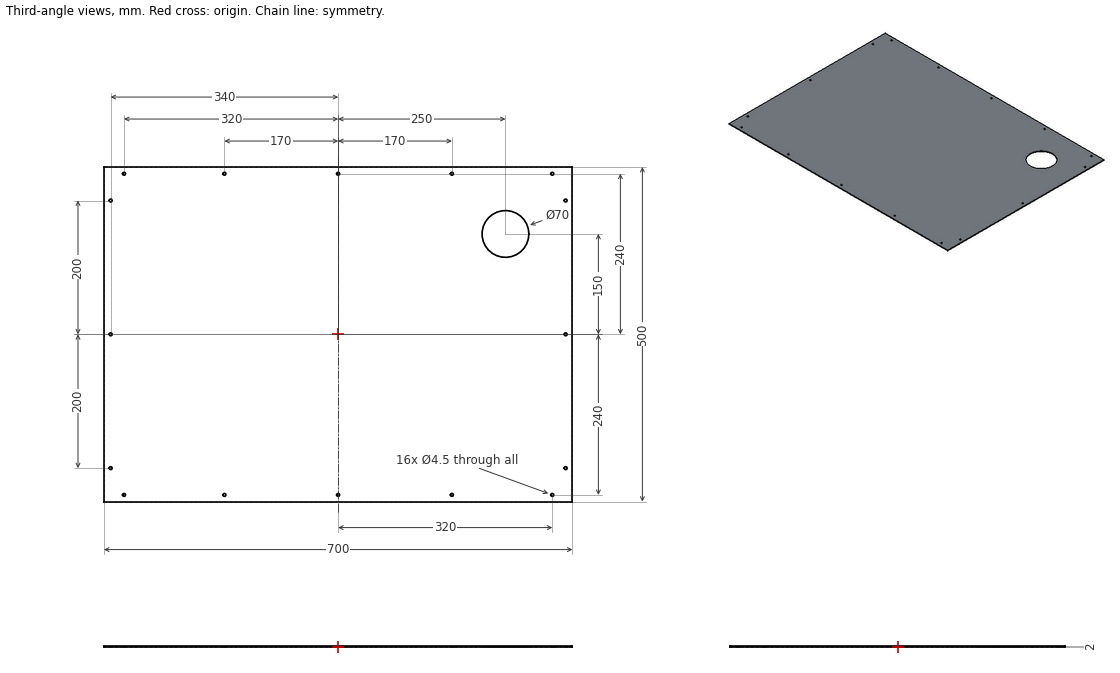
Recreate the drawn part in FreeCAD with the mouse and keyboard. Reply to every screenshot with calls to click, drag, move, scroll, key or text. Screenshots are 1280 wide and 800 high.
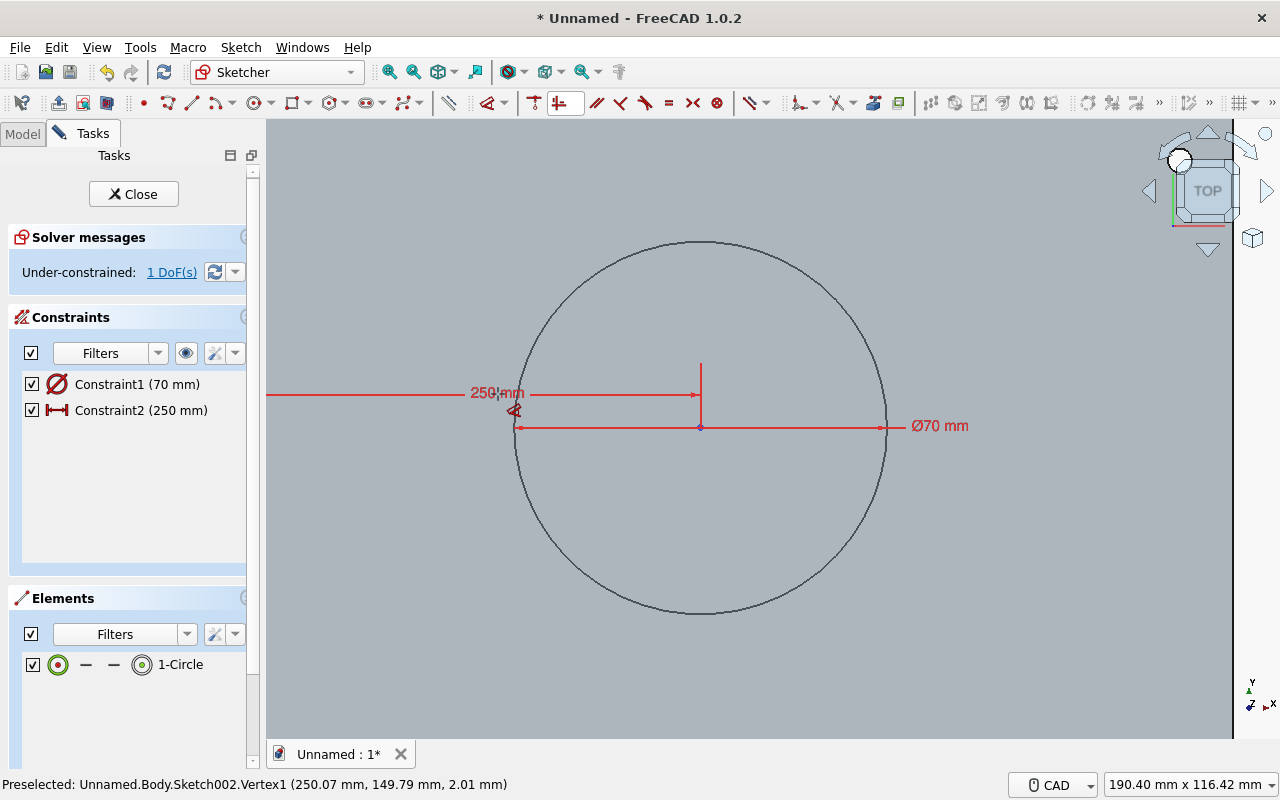
click(701, 428)
click(735, 569)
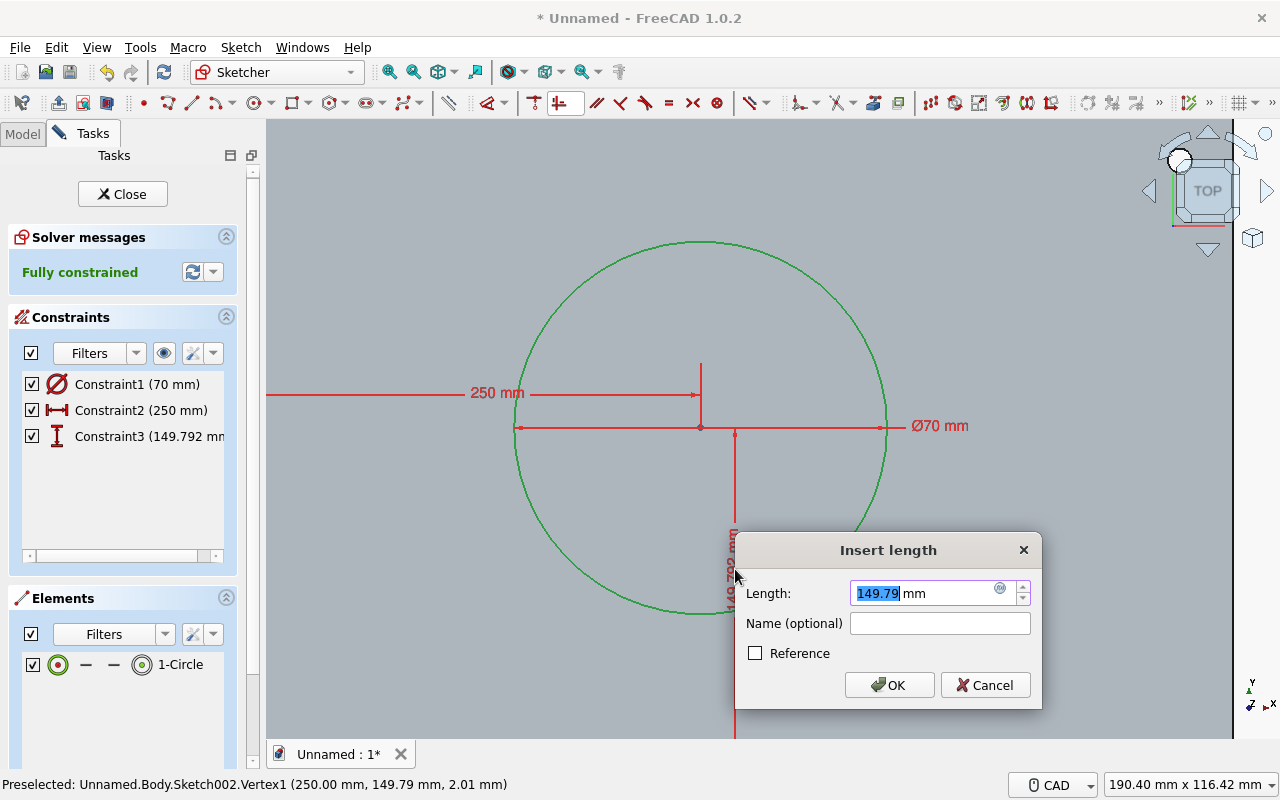
text(150)
key(Return)
key(Escape)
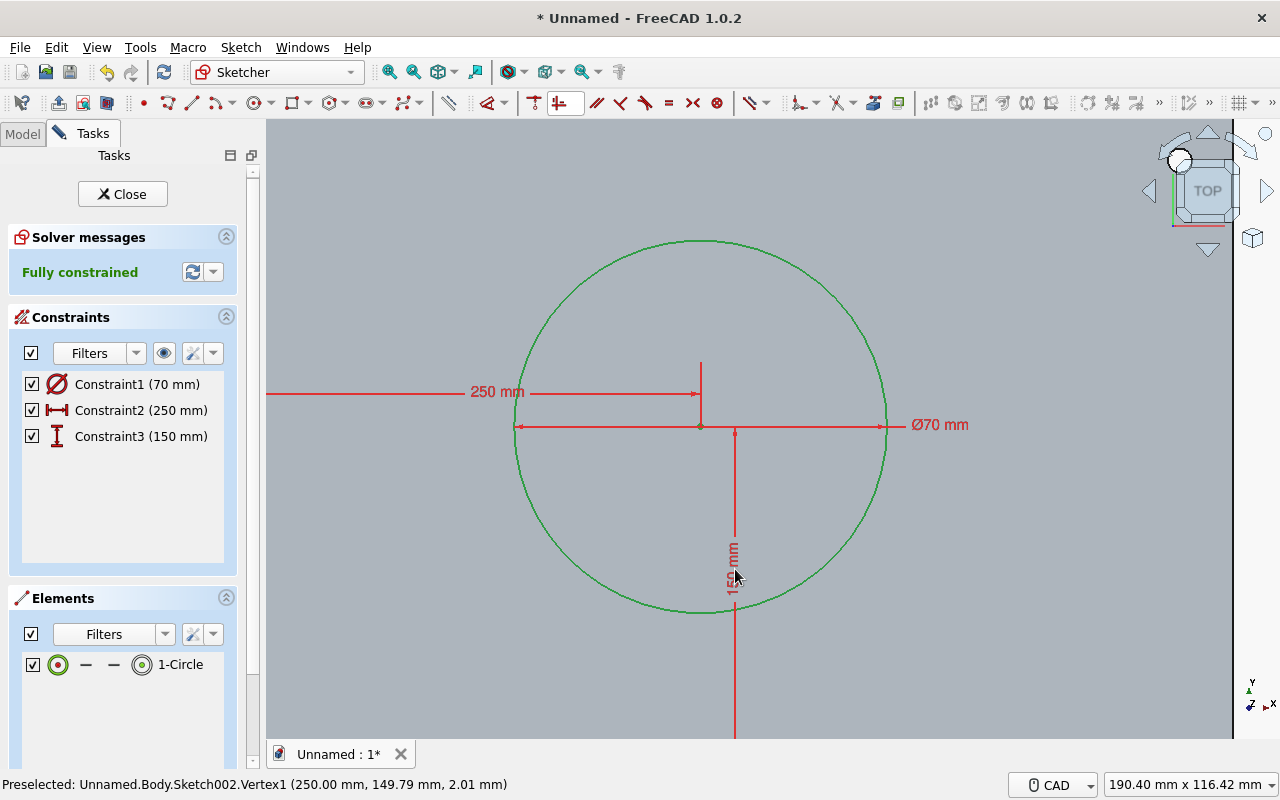
click(123, 194)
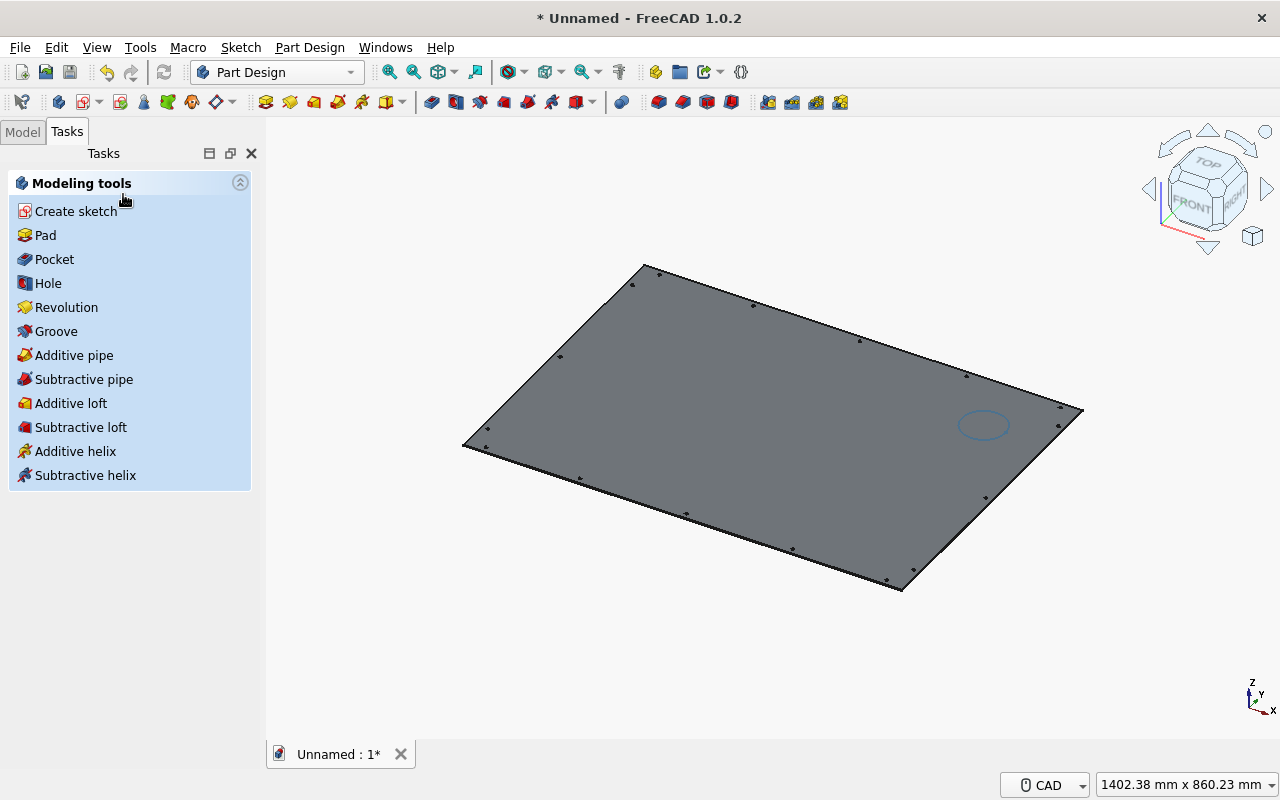
click(432, 102)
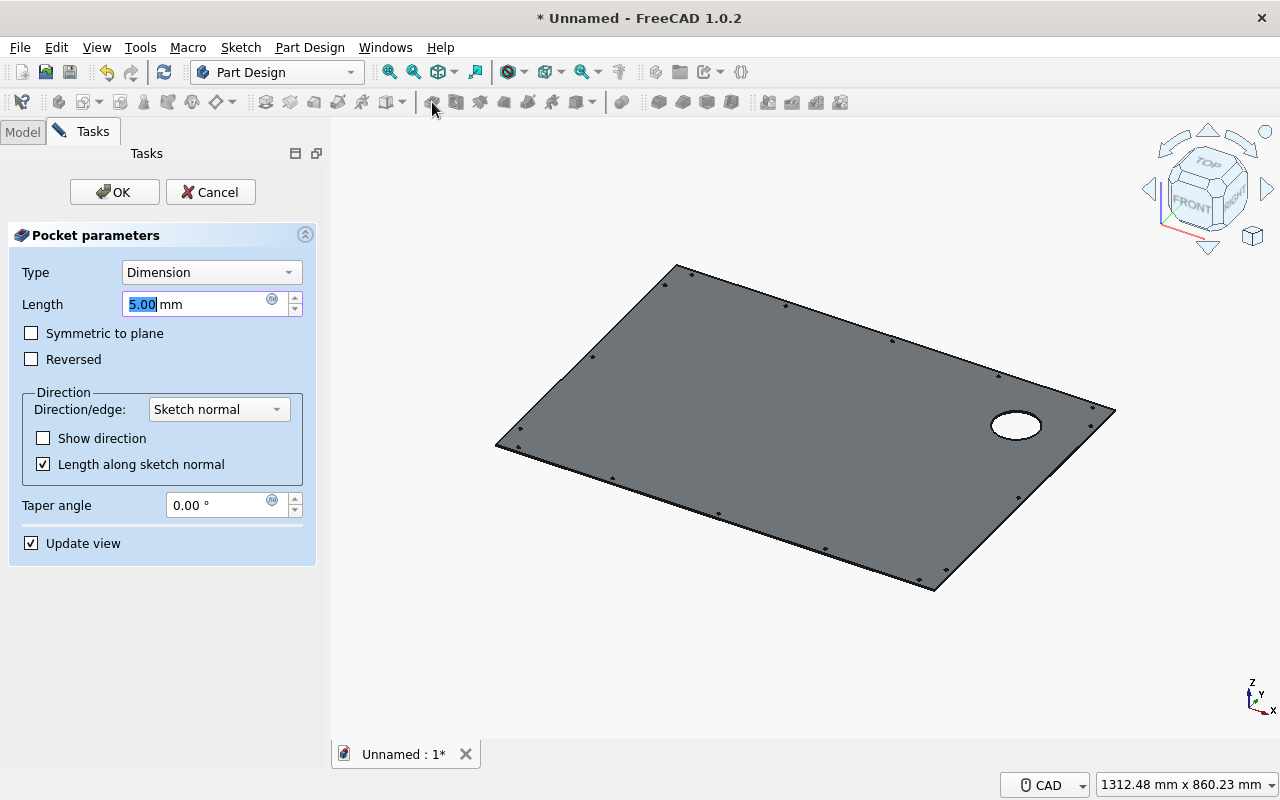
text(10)
key(Tab)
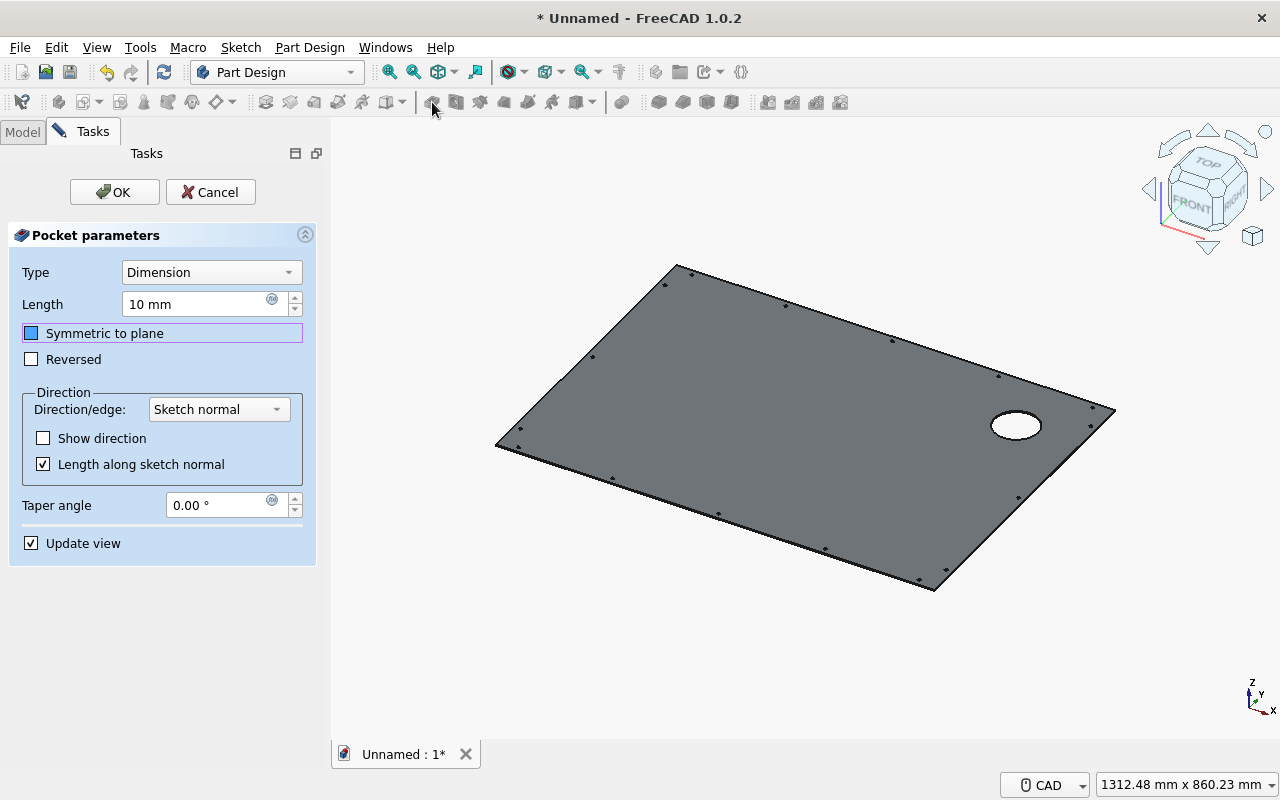
click(115, 192)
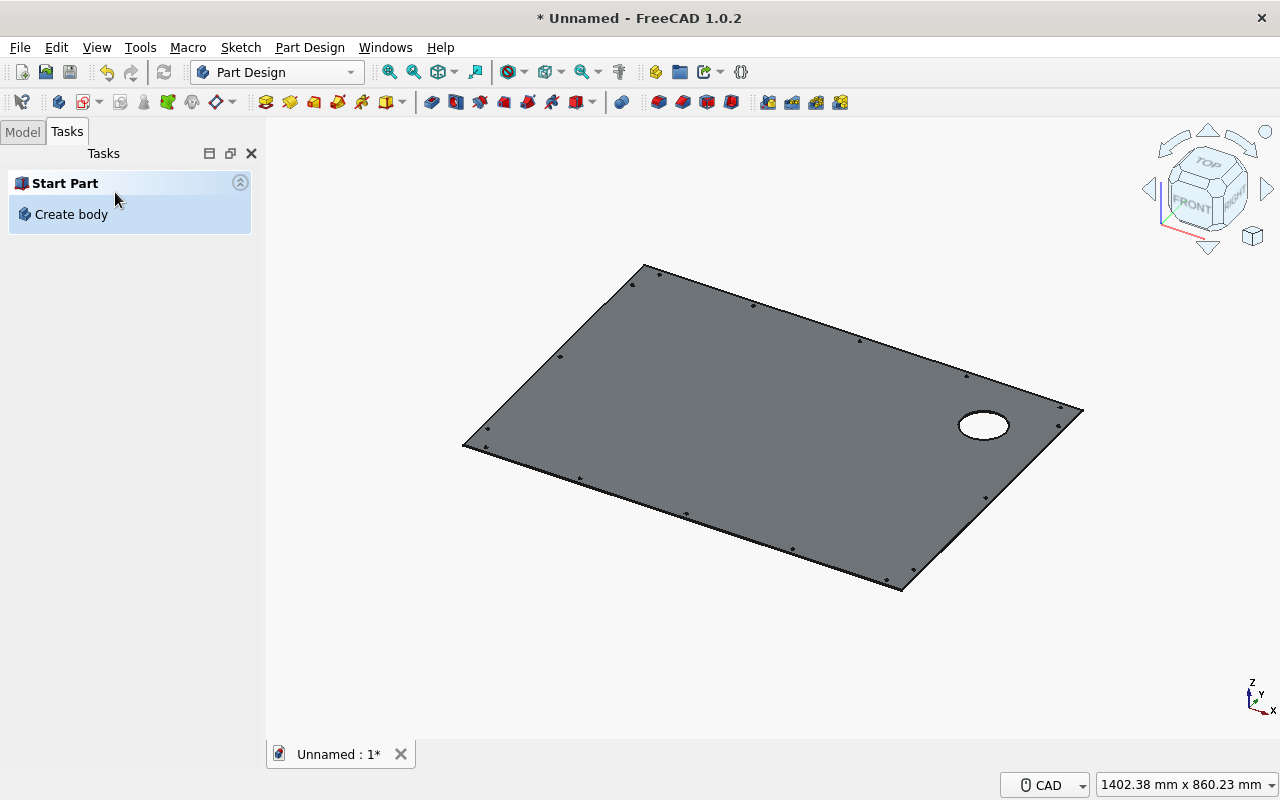
key(0)